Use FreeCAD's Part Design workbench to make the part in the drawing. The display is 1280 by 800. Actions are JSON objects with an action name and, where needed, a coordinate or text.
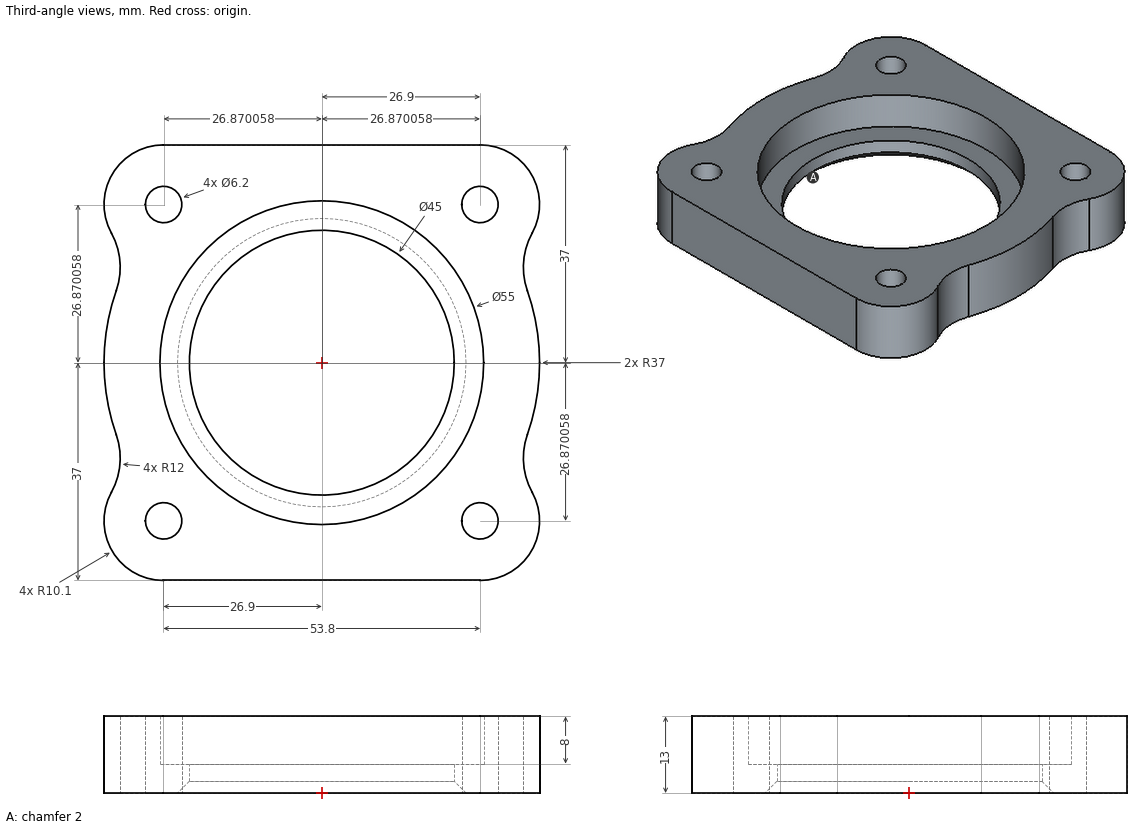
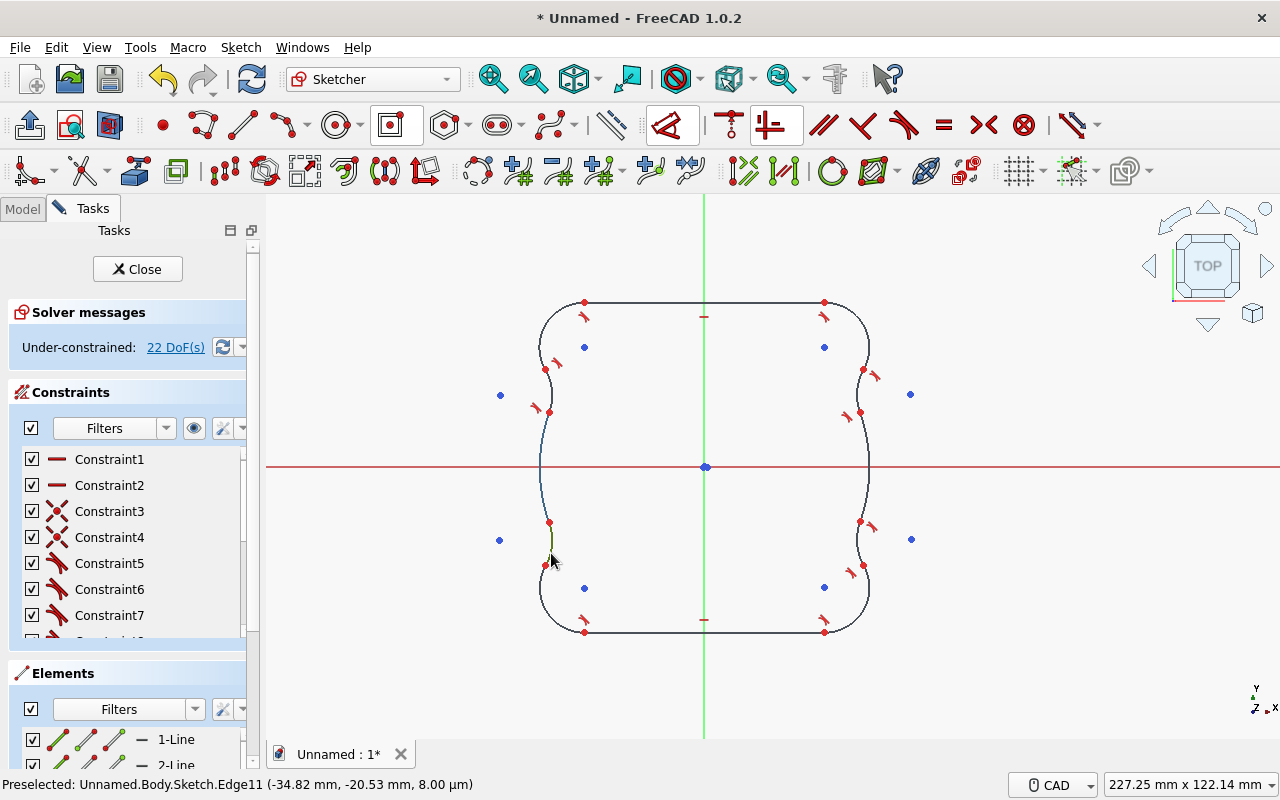
{"action": "key", "text": "t"}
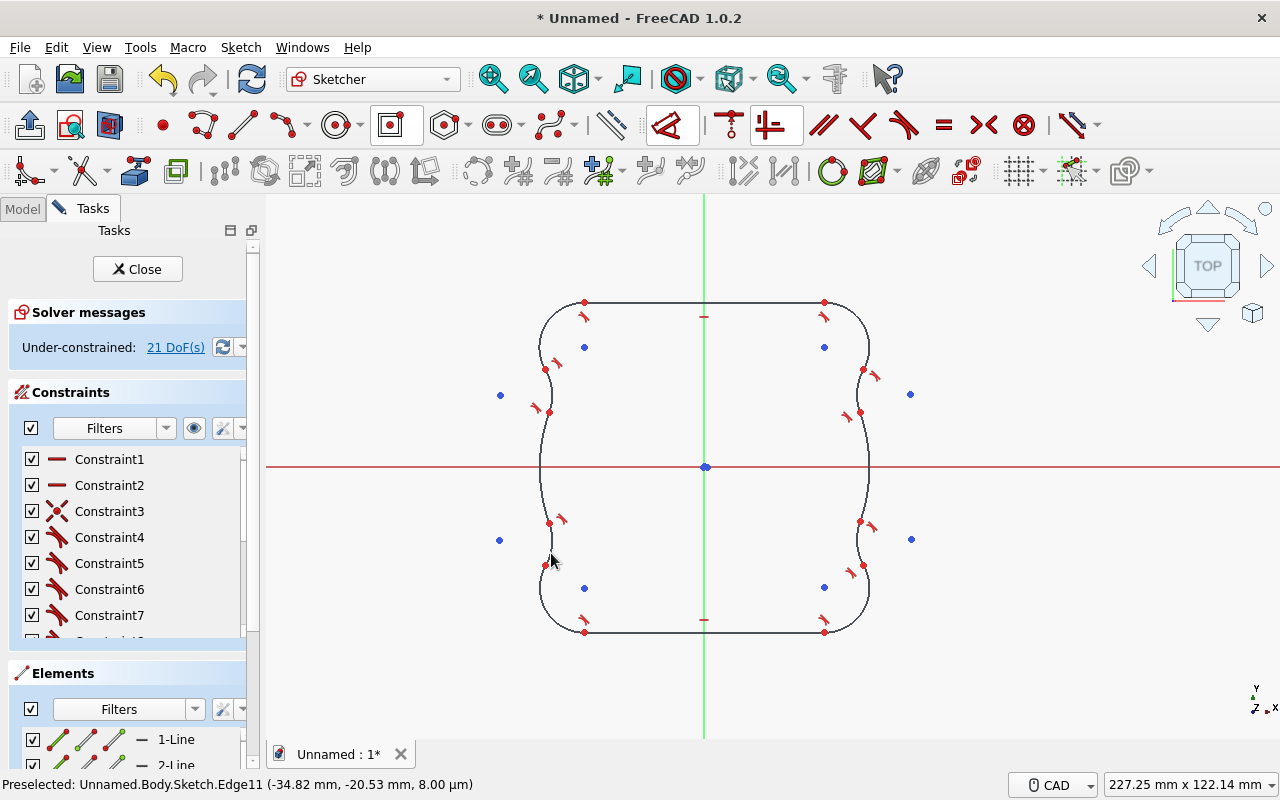
{"action": "left_click", "coordinate": [551, 554]}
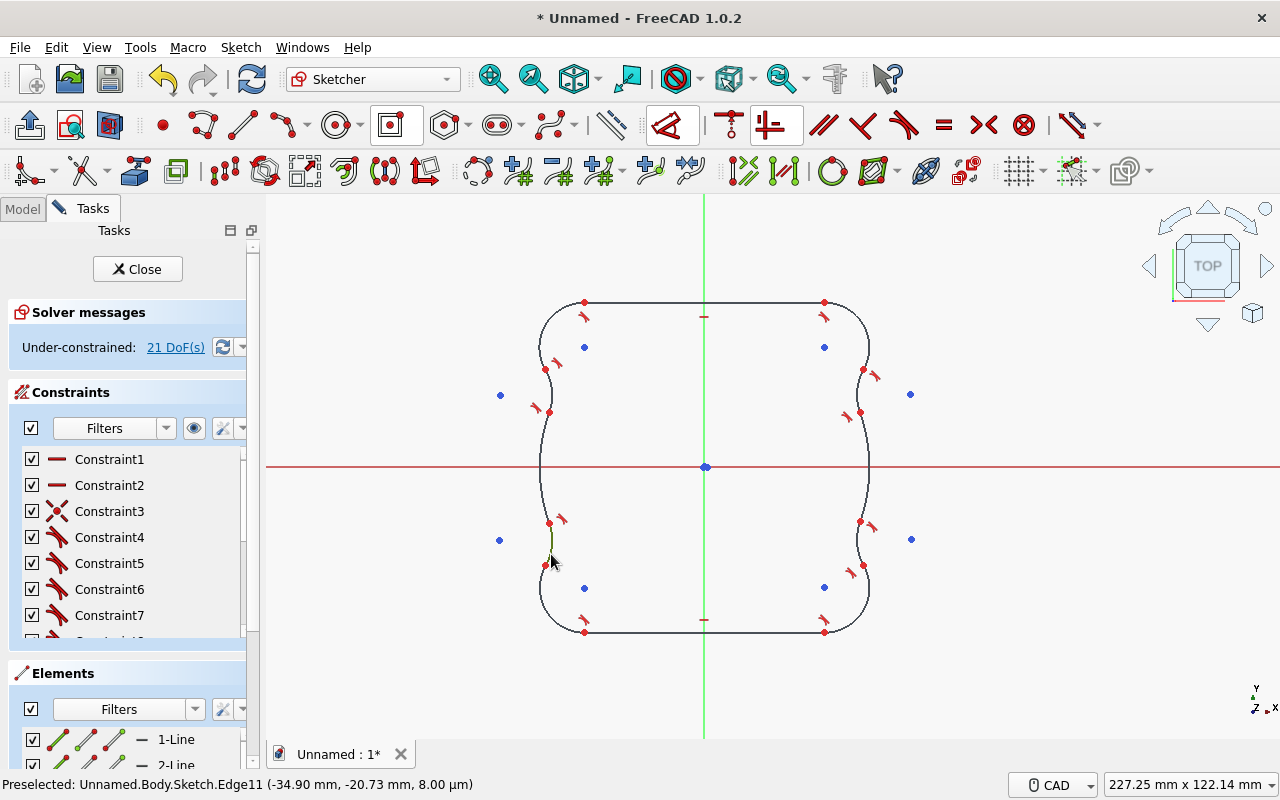
{"action": "left_click", "coordinate": [540, 593]}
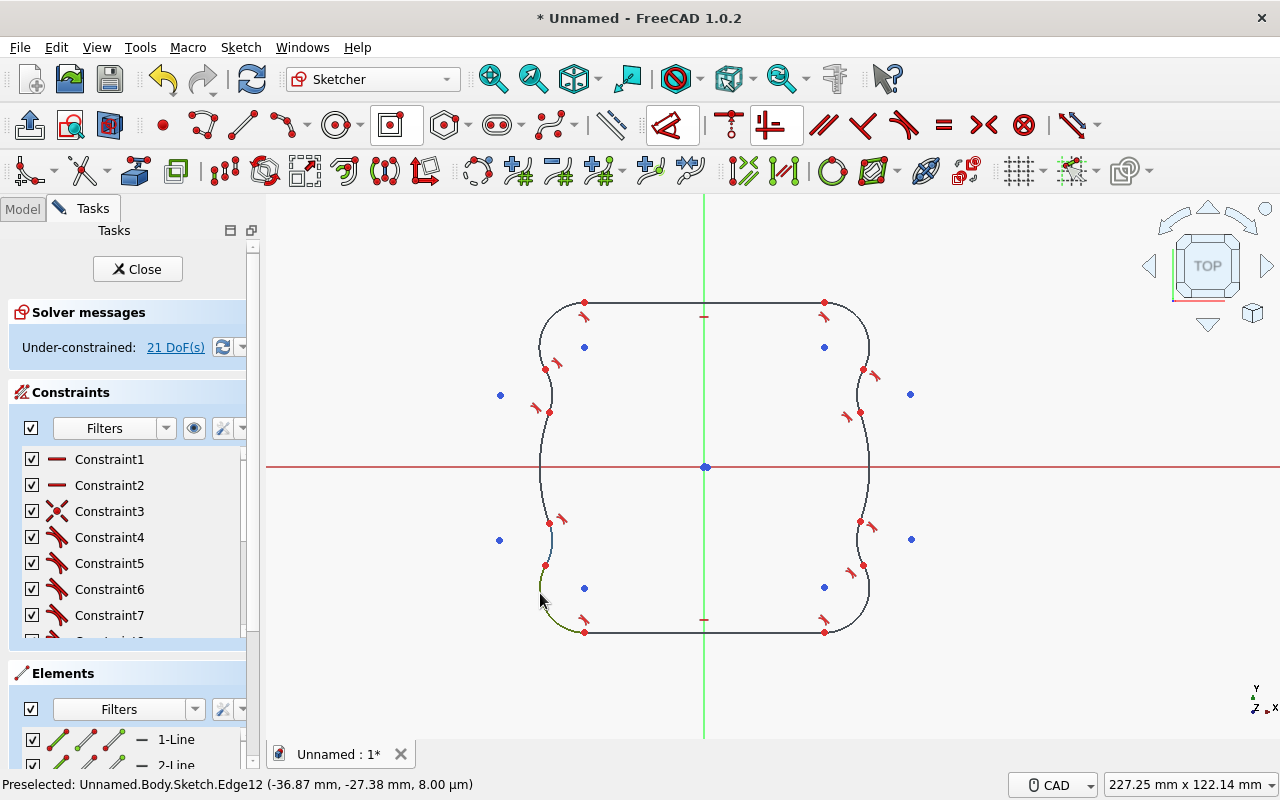
{"action": "left_click", "coordinate": [904, 126]}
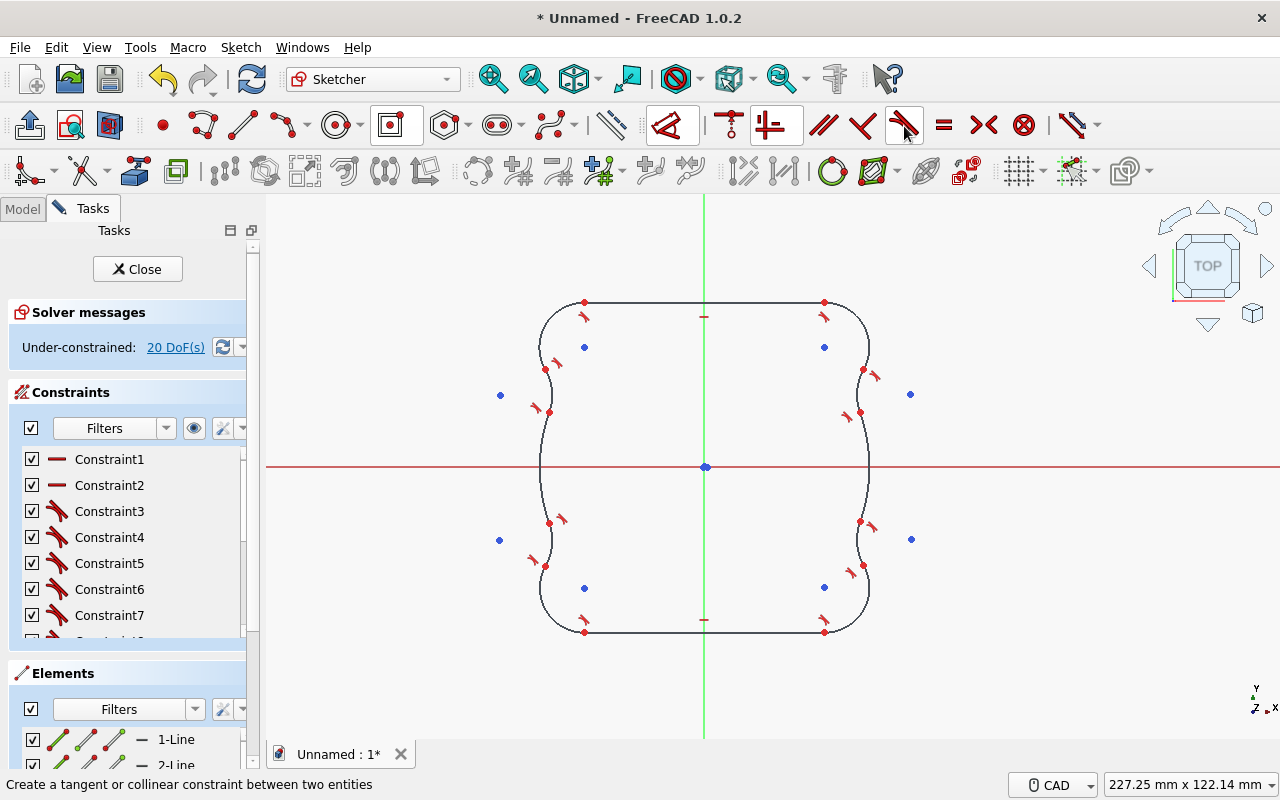
{"action": "left_click", "coordinate": [868, 489]}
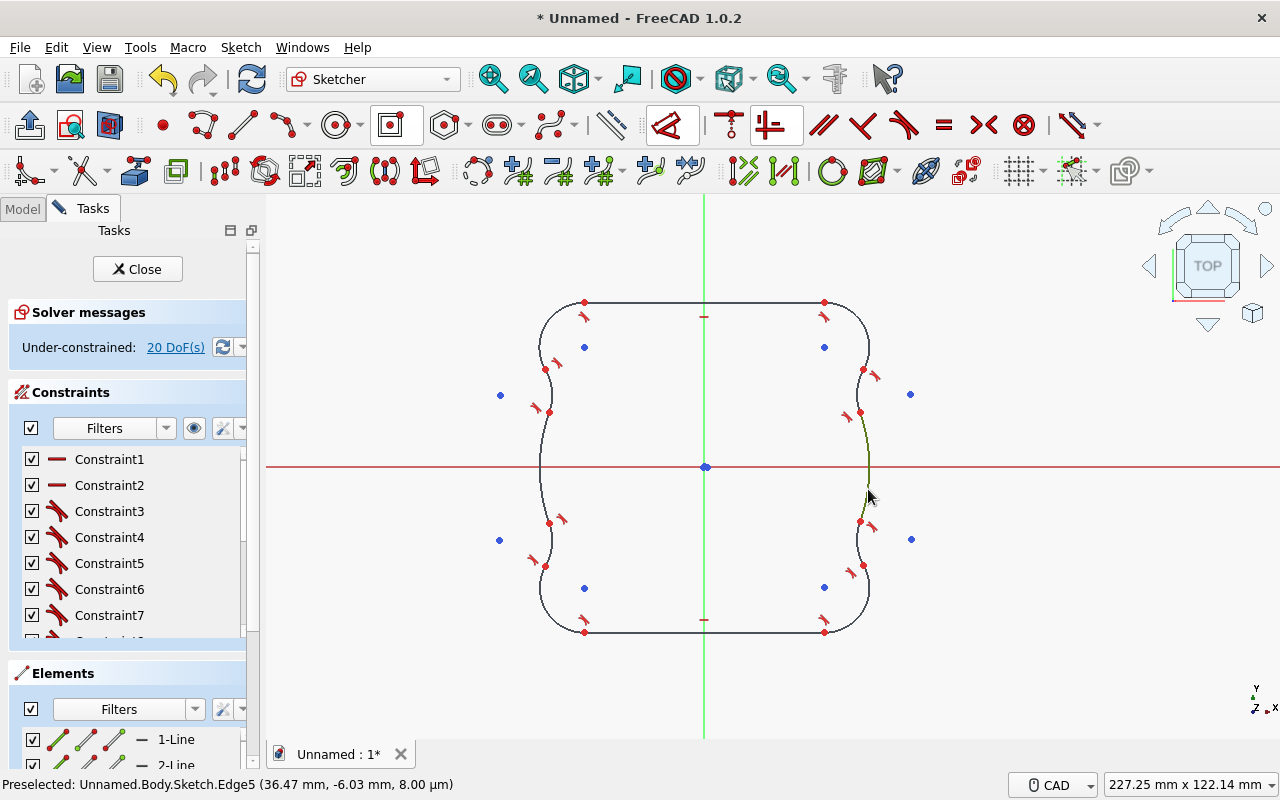
{"action": "left_click", "coordinate": [541, 445]}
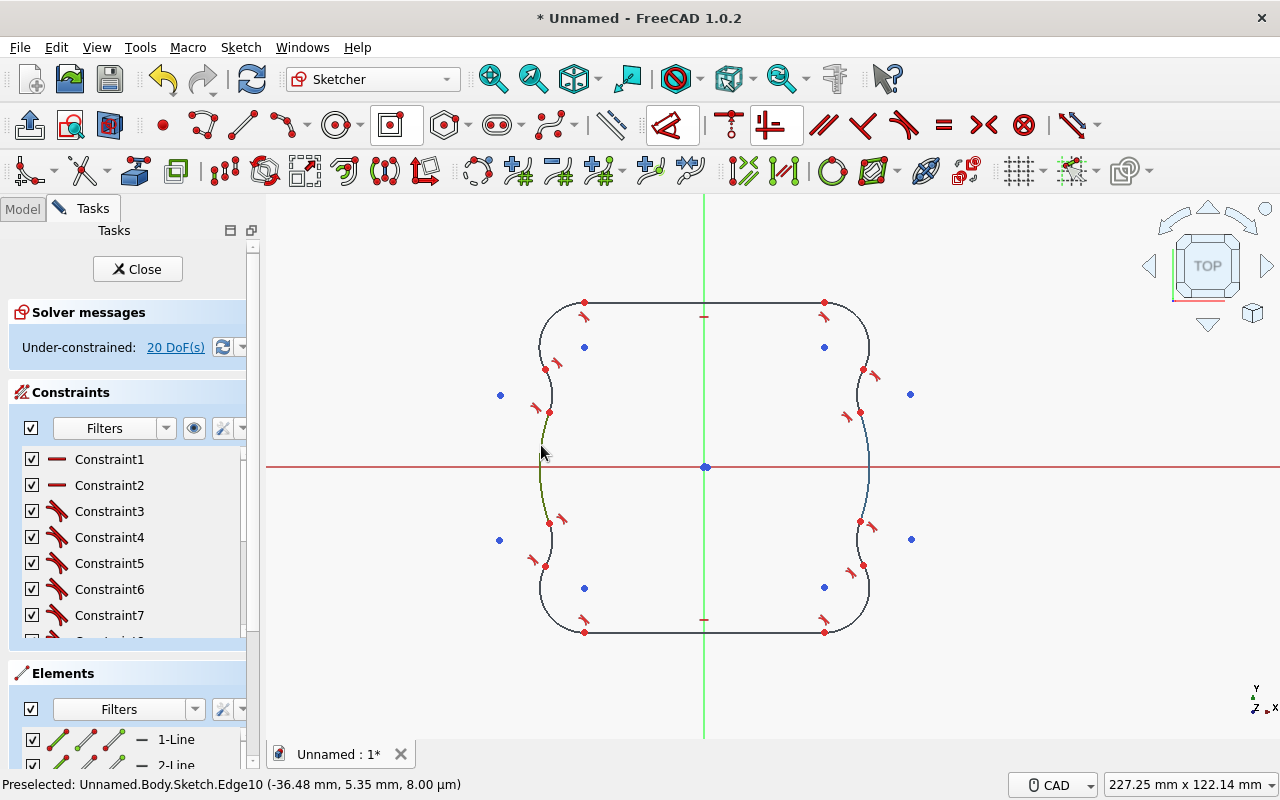
{"action": "left_click", "coordinate": [730, 126]}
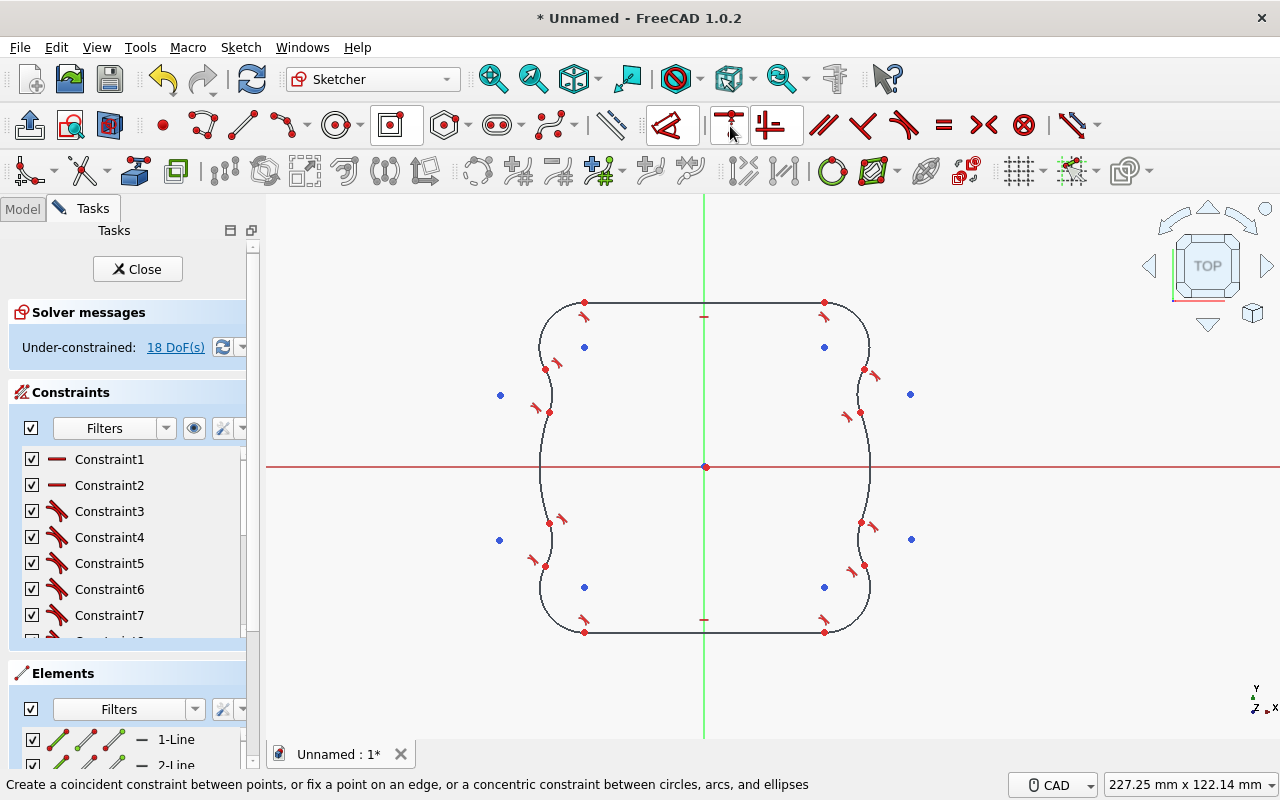
{"action": "left_click_drag", "start_coordinate": [694, 457], "coordinate": [716, 478]}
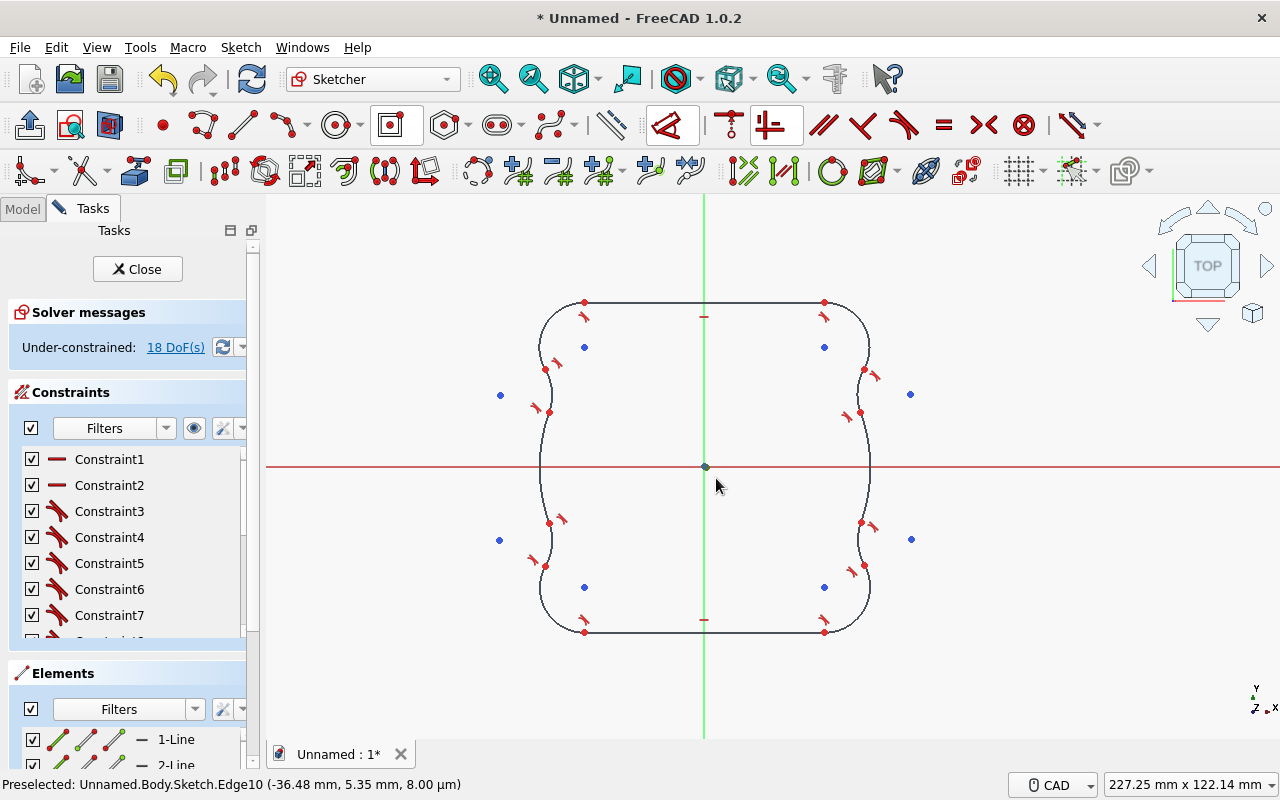
{"action": "key", "text": "c"}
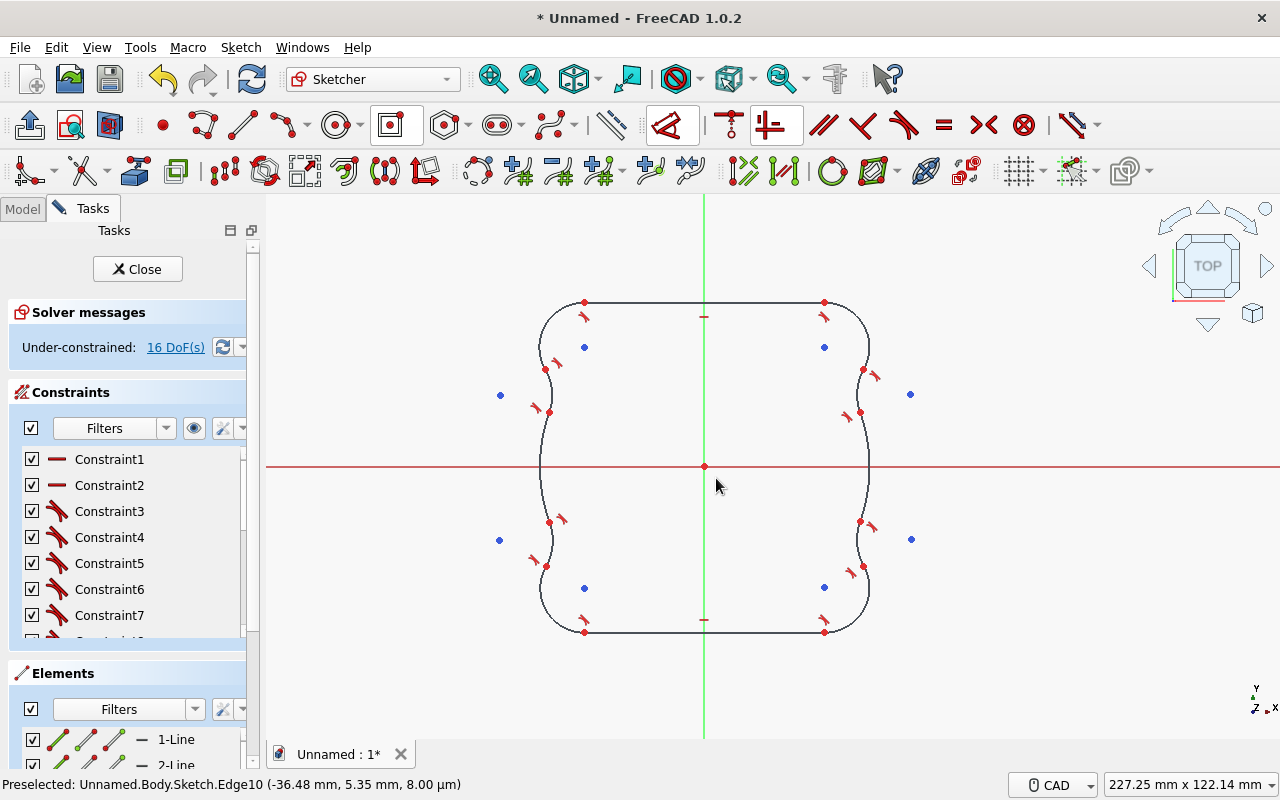
{"action": "left_click", "coordinate": [857, 535]}